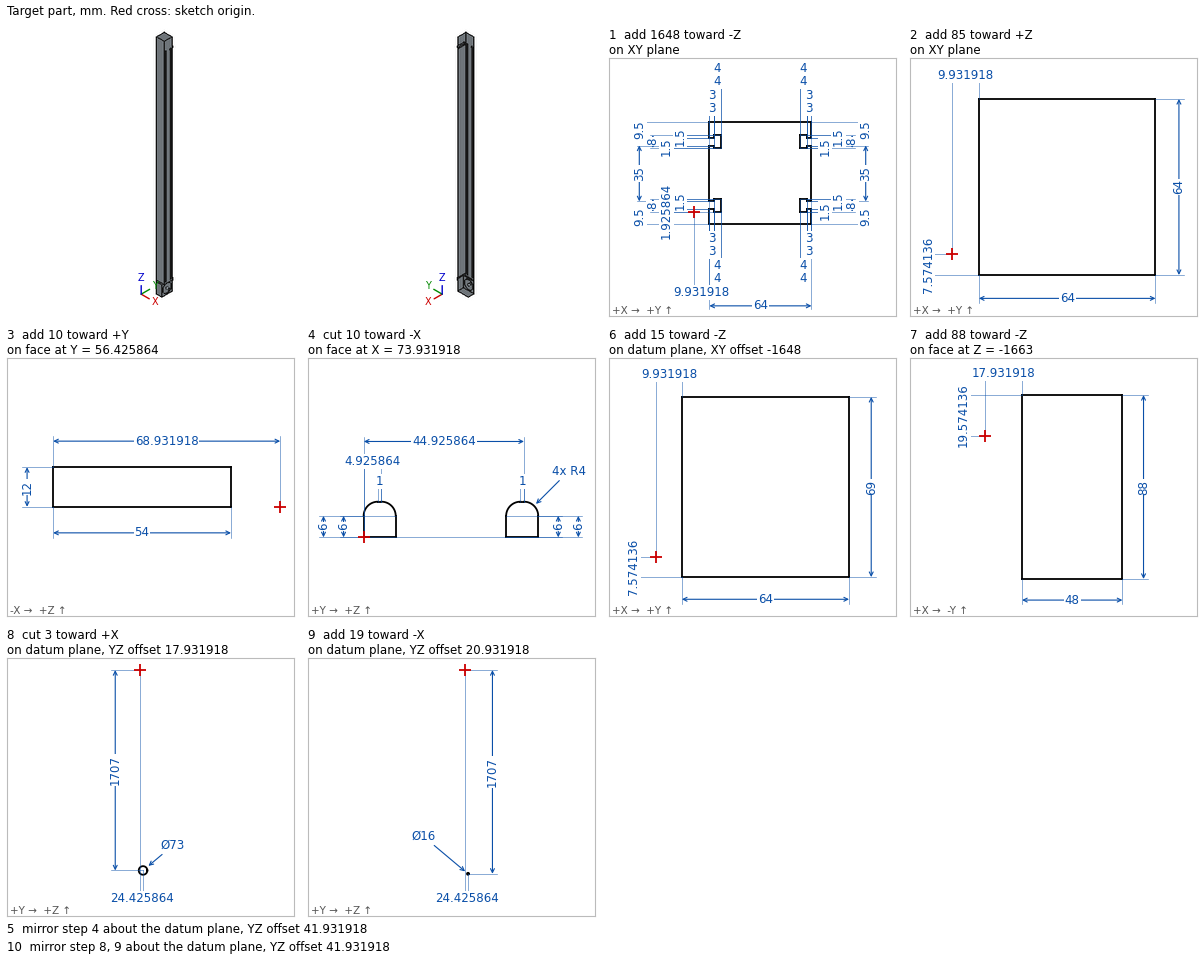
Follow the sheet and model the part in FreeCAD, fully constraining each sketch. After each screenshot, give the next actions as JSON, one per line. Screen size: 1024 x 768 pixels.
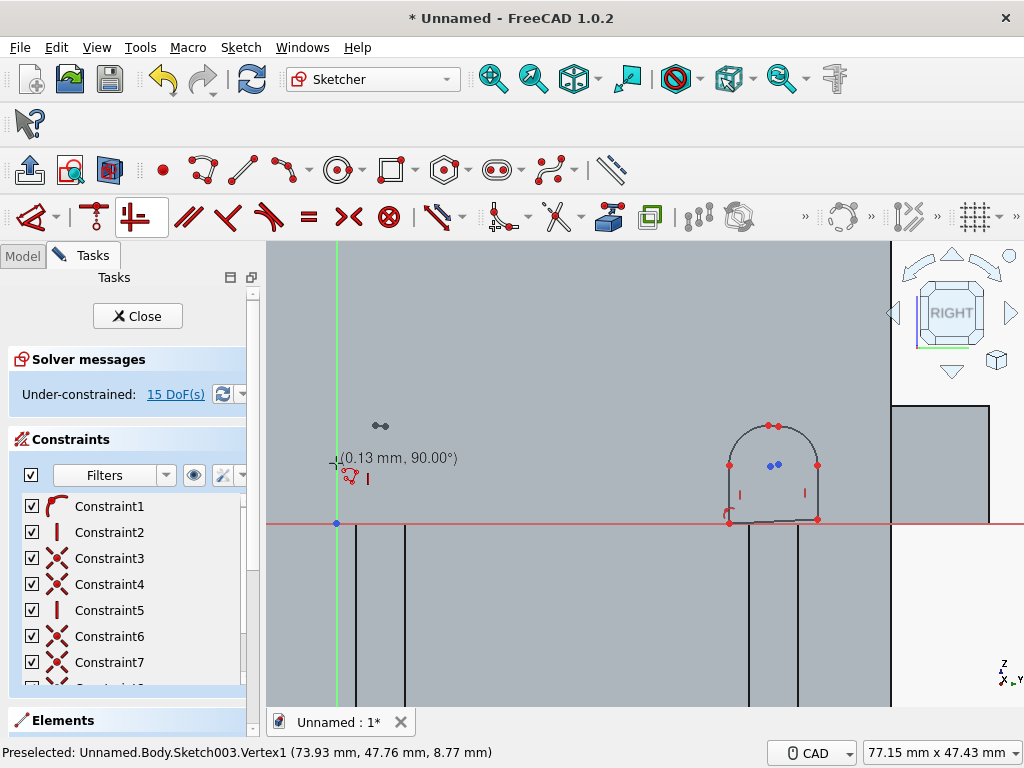
{"action": "scroll", "coordinate": [336, 524], "scroll_direction": "up", "scroll_amount": 16}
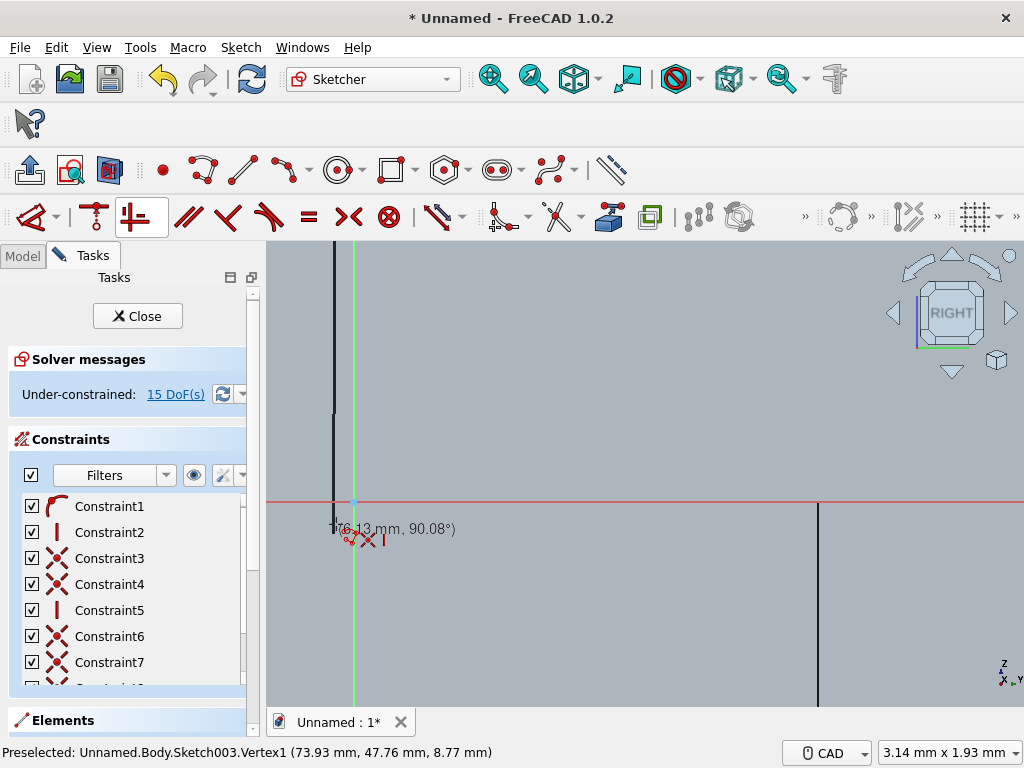
{"action": "left_click", "coordinate": [336, 502]}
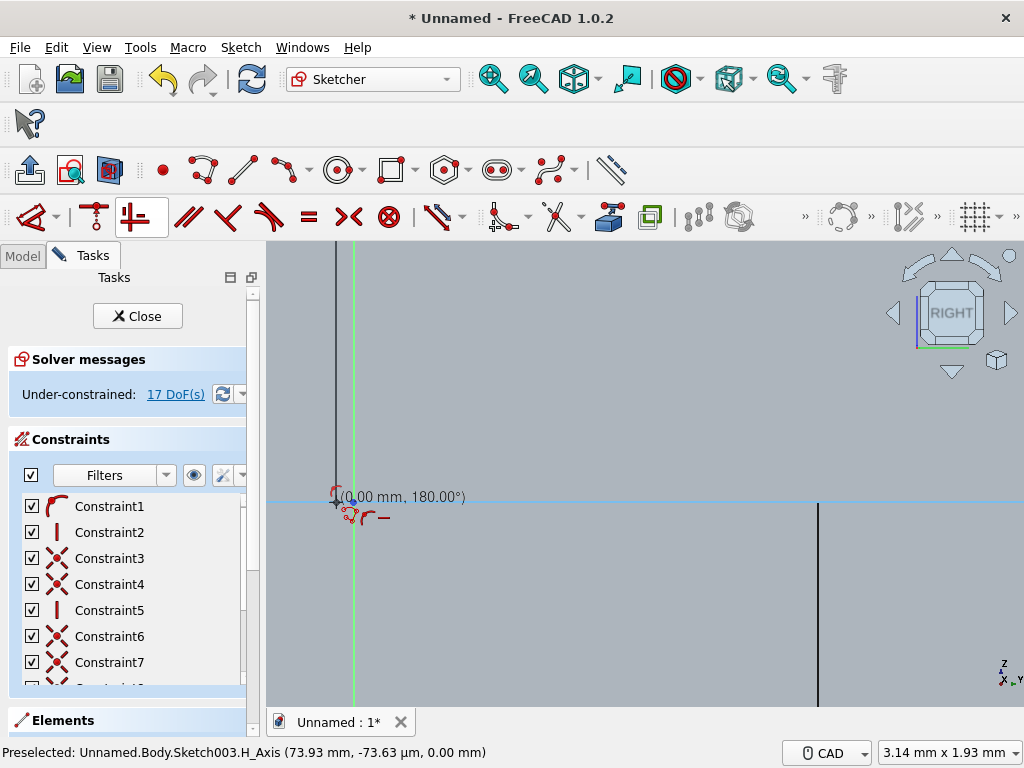
{"action": "scroll", "coordinate": [336, 524], "scroll_direction": "down", "scroll_amount": 16}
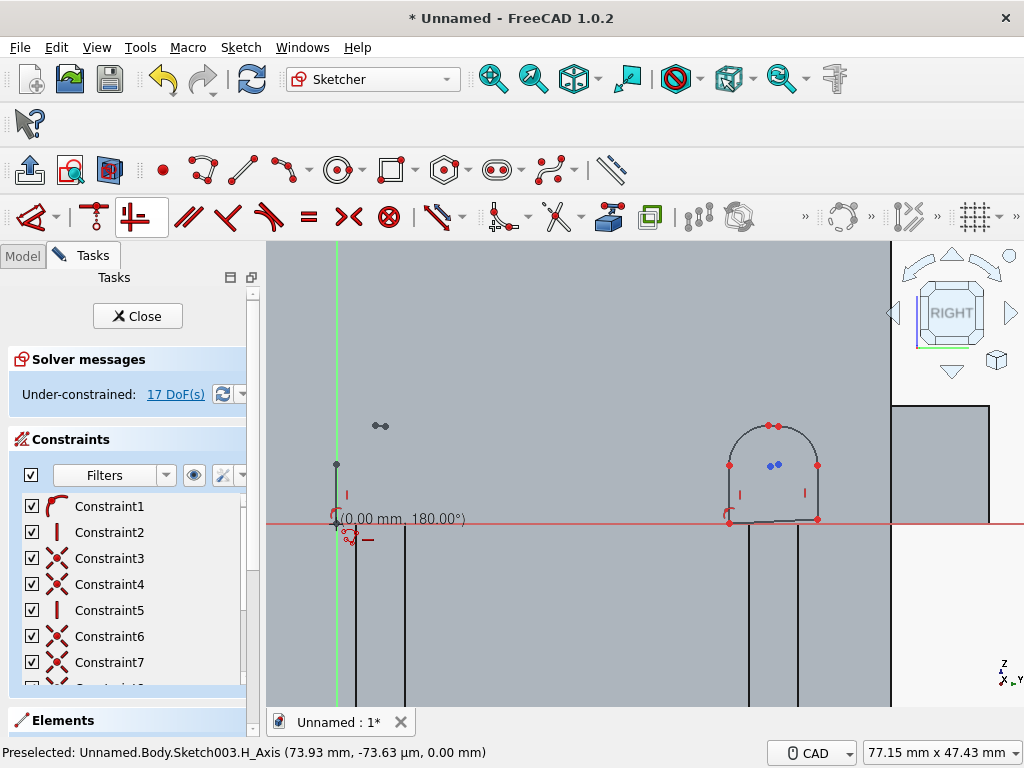
{"action": "left_click", "coordinate": [425, 515]}
{"action": "left_click", "coordinate": [425, 465]}
{"action": "right_click", "coordinate": [425, 465]}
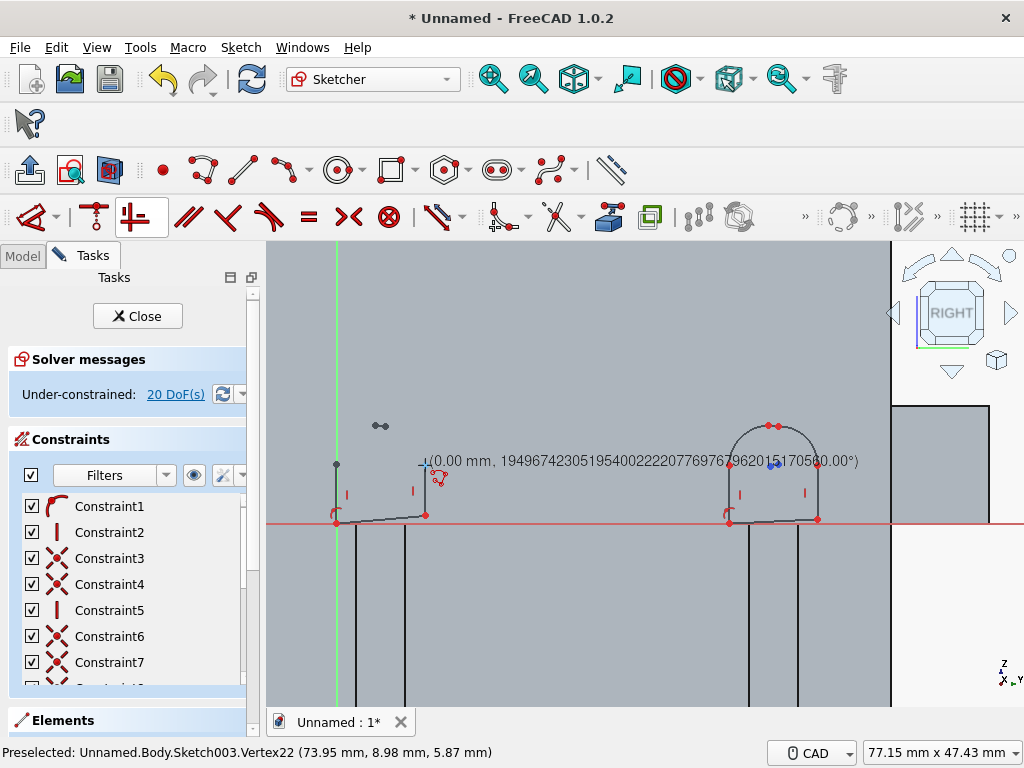
{"action": "left_click", "coordinate": [284, 170]}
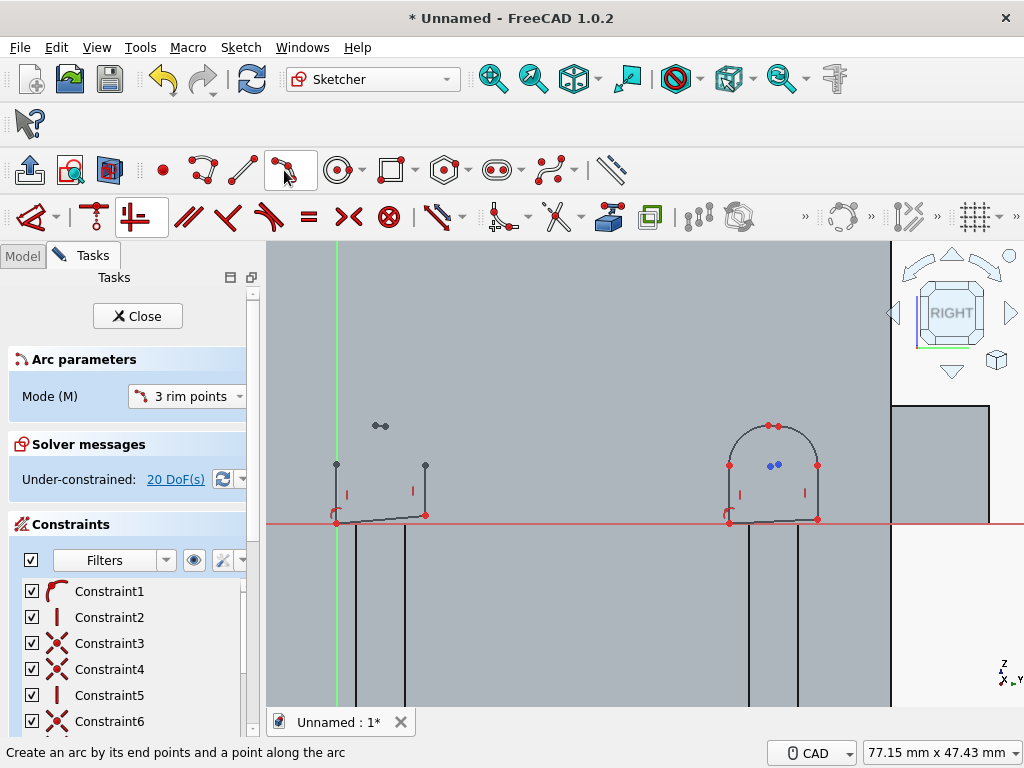
{"action": "scroll", "coordinate": [375, 425], "scroll_direction": "up", "scroll_amount": 6}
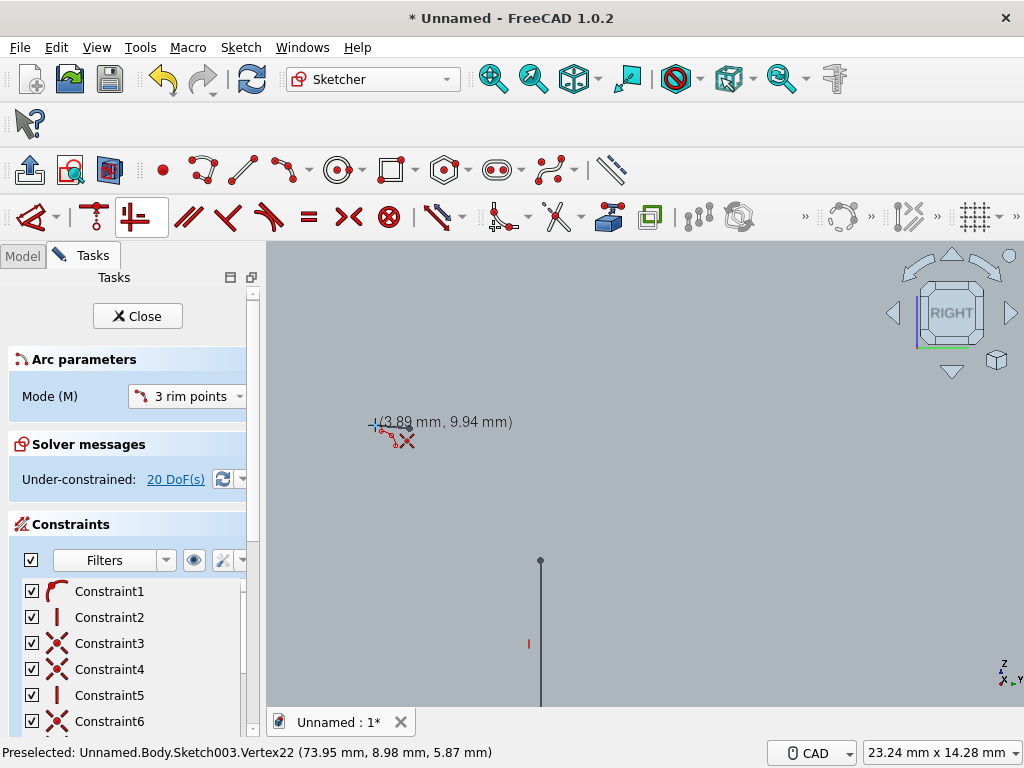
{"action": "left_click", "coordinate": [375, 425]}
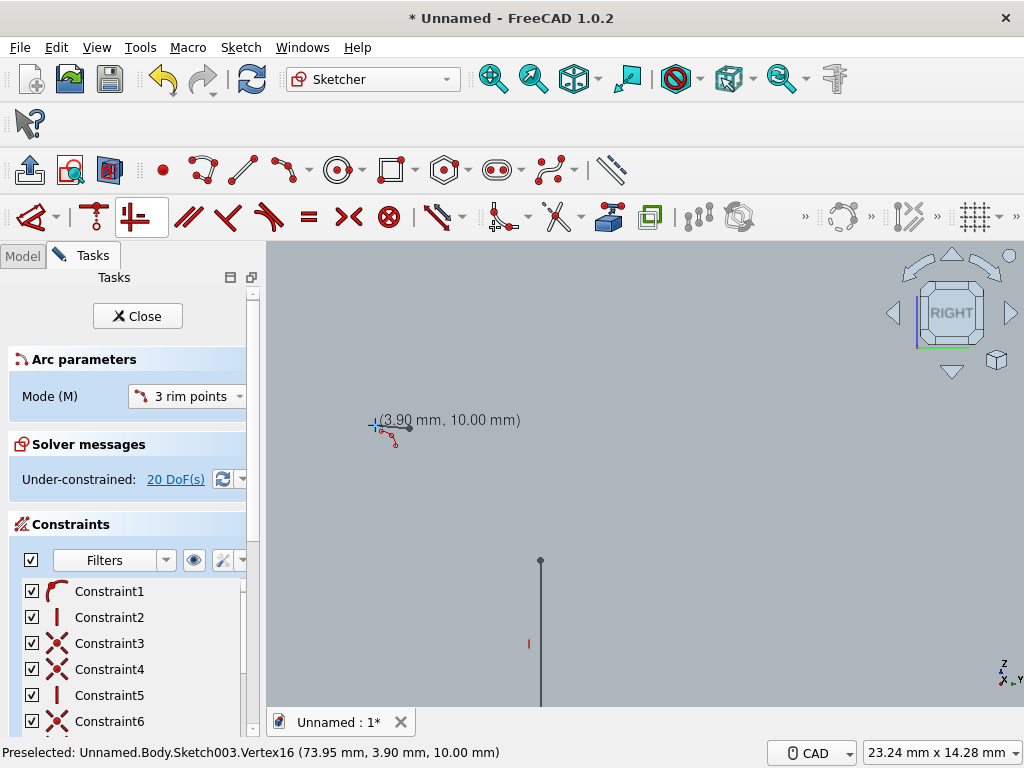
{"action": "scroll", "coordinate": [423, 436], "scroll_direction": "down", "scroll_amount": 7}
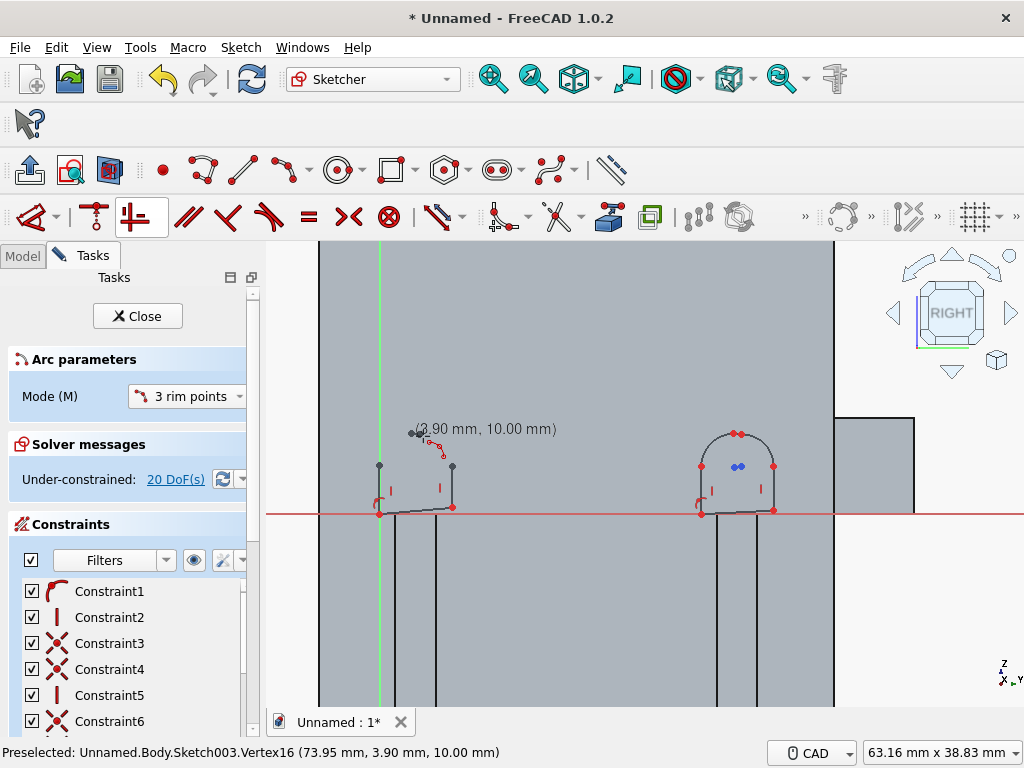
{"action": "scroll", "coordinate": [379, 466], "scroll_direction": "up", "scroll_amount": 17}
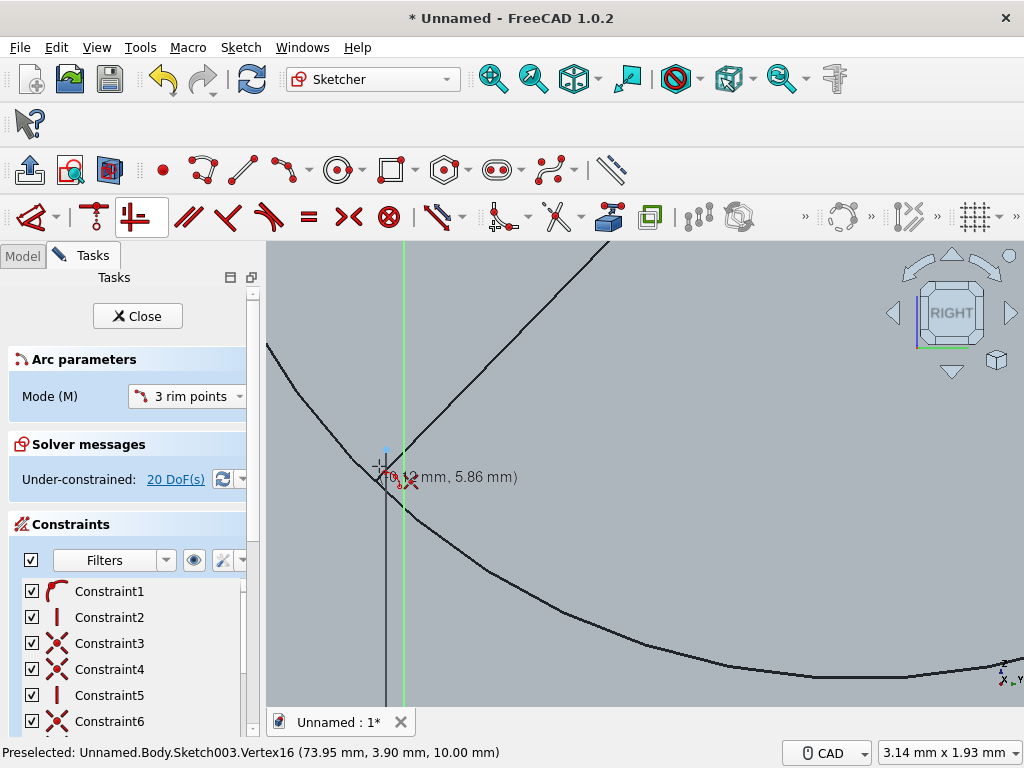
{"action": "left_click", "coordinate": [386, 450]}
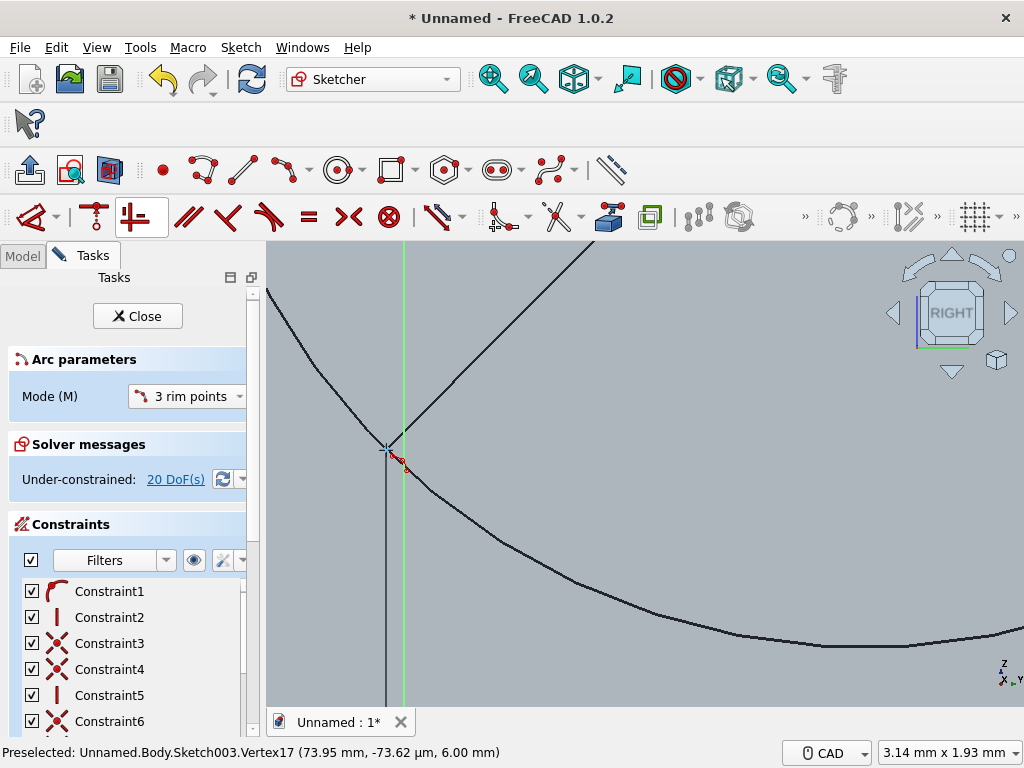
{"action": "scroll", "coordinate": [334, 465], "scroll_direction": "down", "scroll_amount": 16}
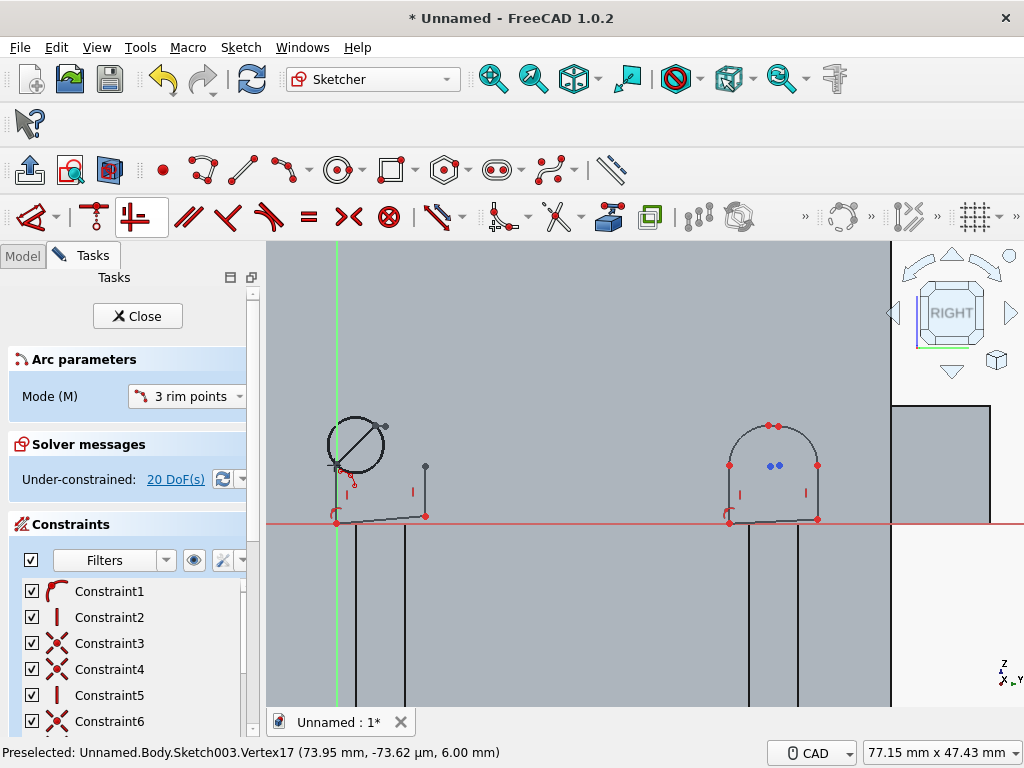
{"action": "scroll", "coordinate": [352, 433], "scroll_direction": "up", "scroll_amount": 2}